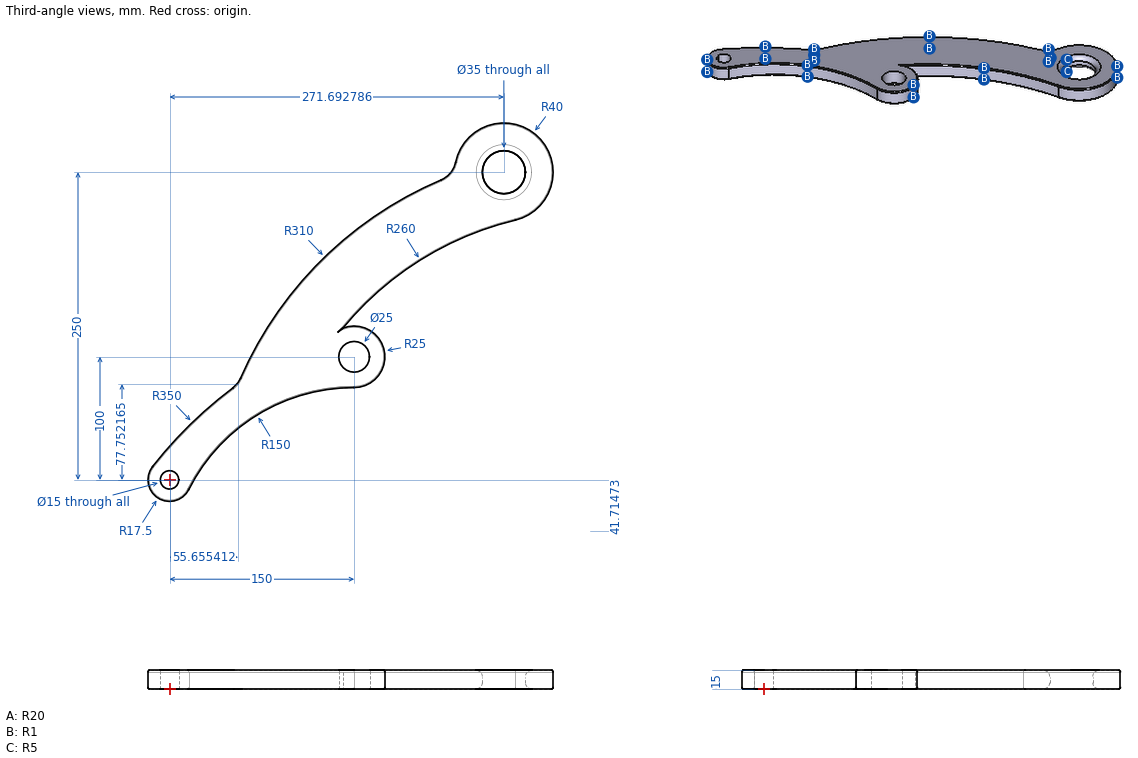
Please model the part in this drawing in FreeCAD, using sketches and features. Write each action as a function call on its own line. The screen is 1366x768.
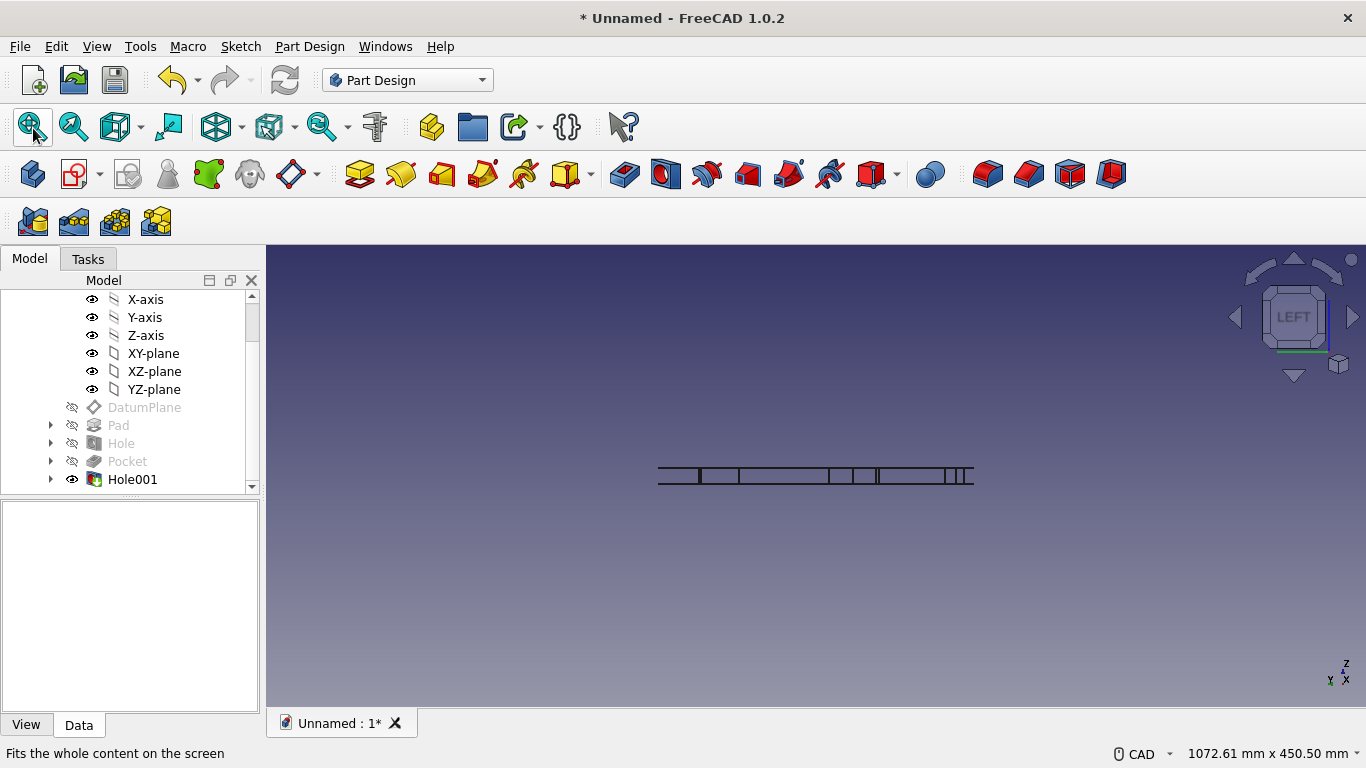
key(0)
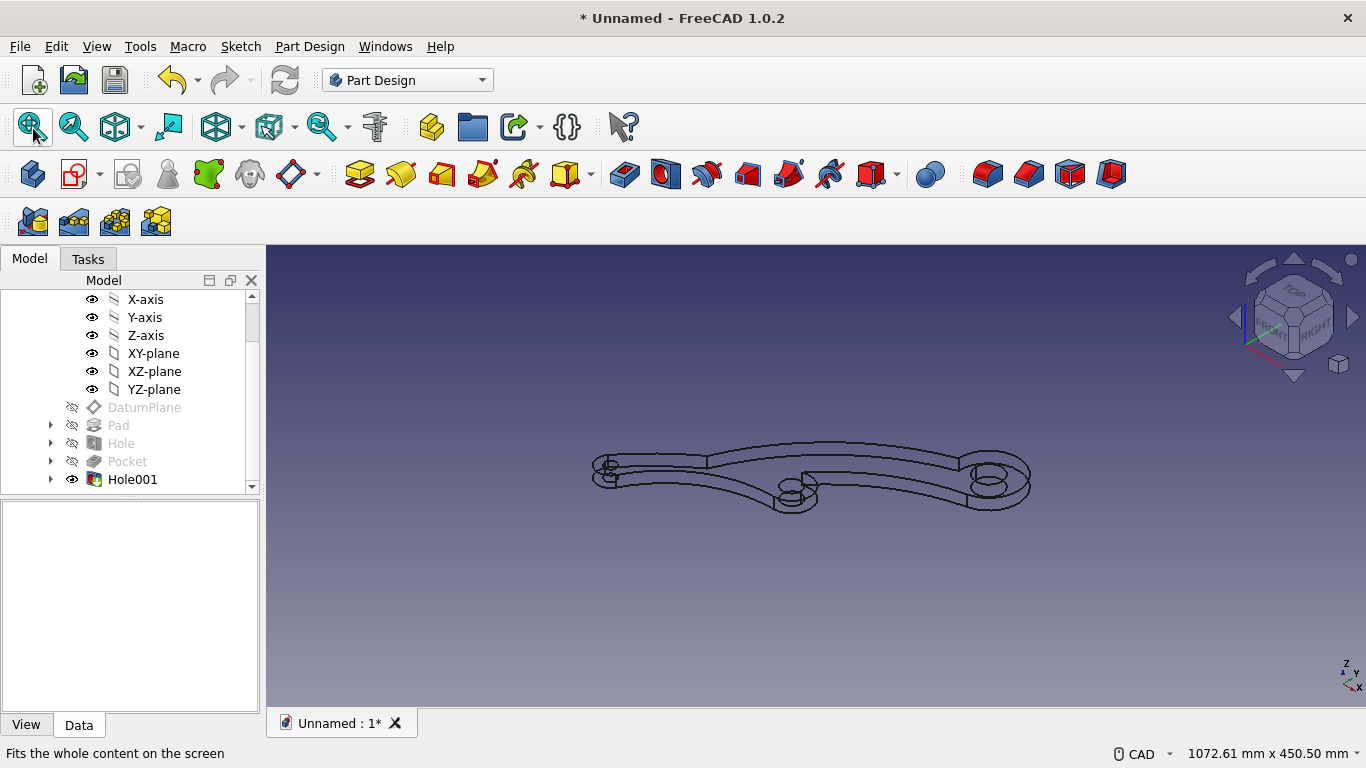
click(707, 461)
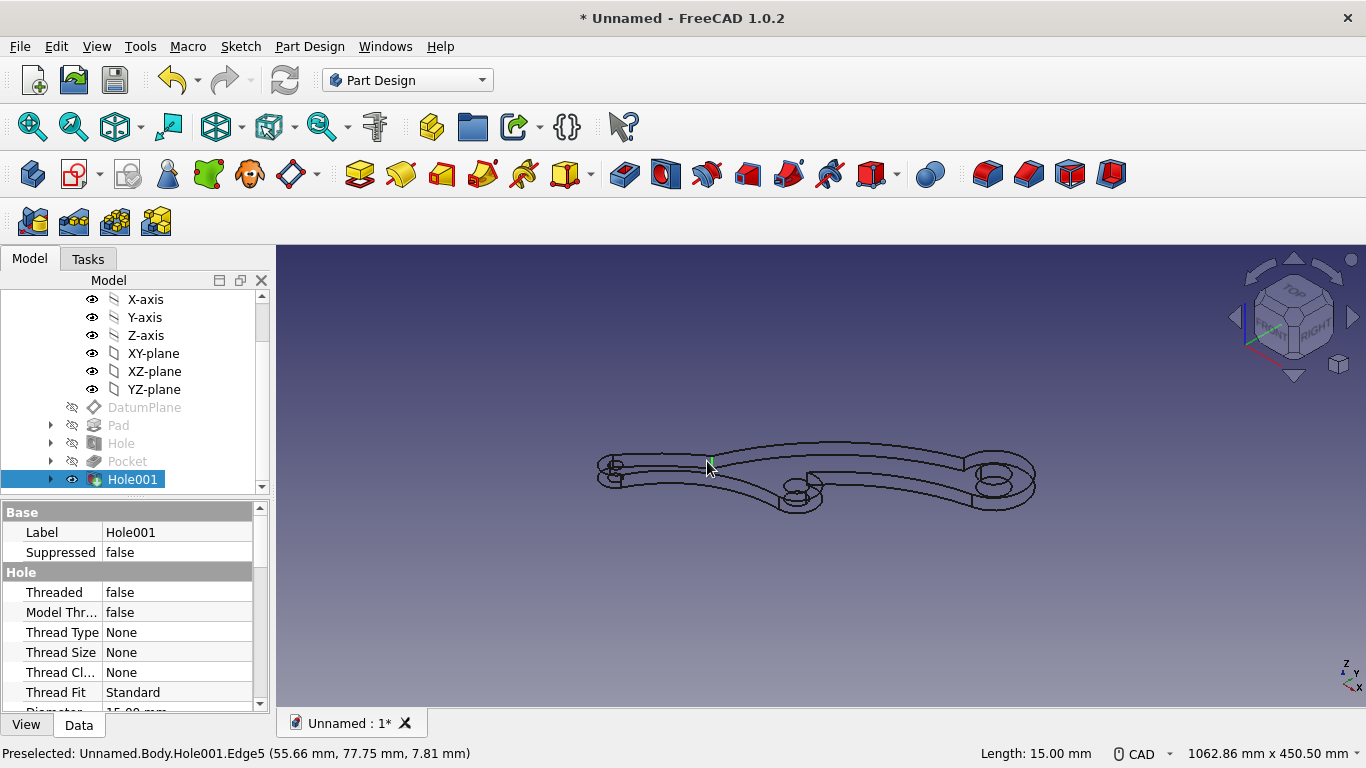
click(964, 464, ctrl)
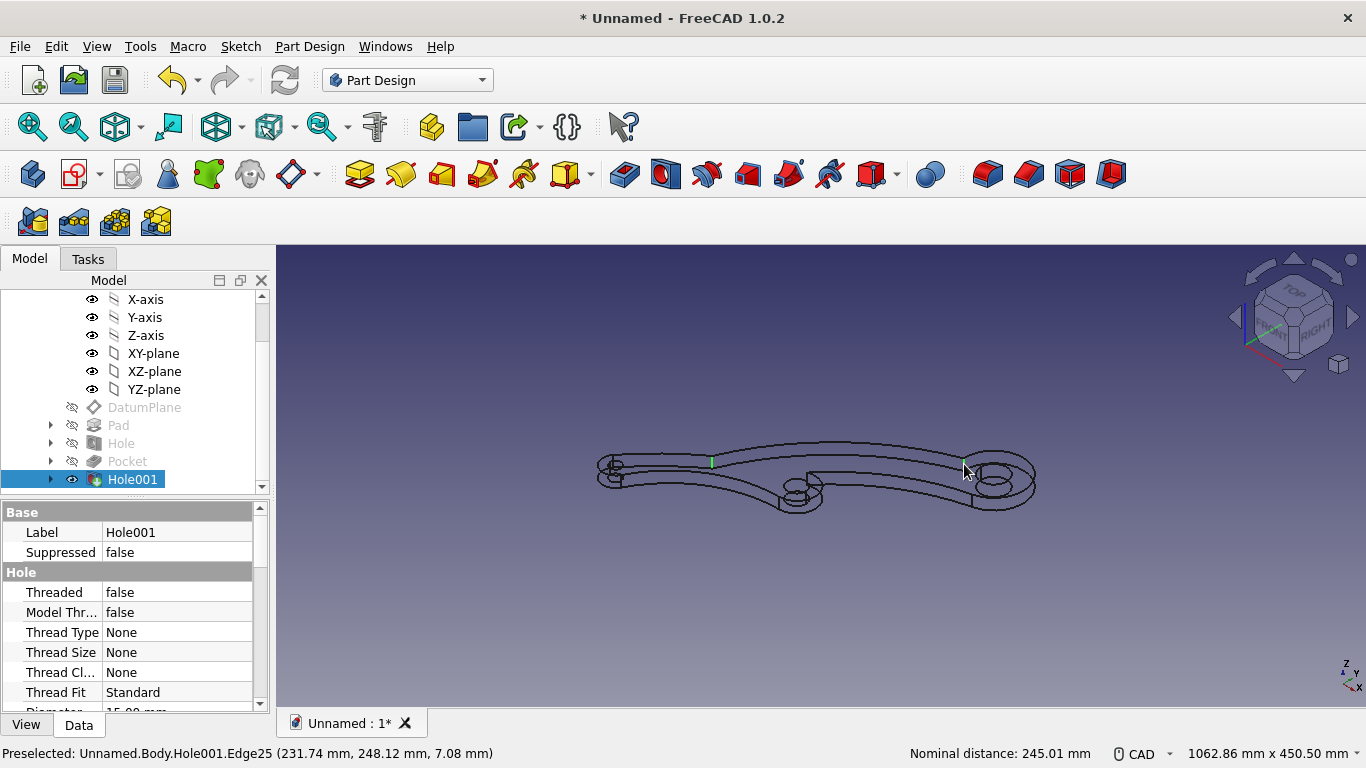
key(v)
key(1)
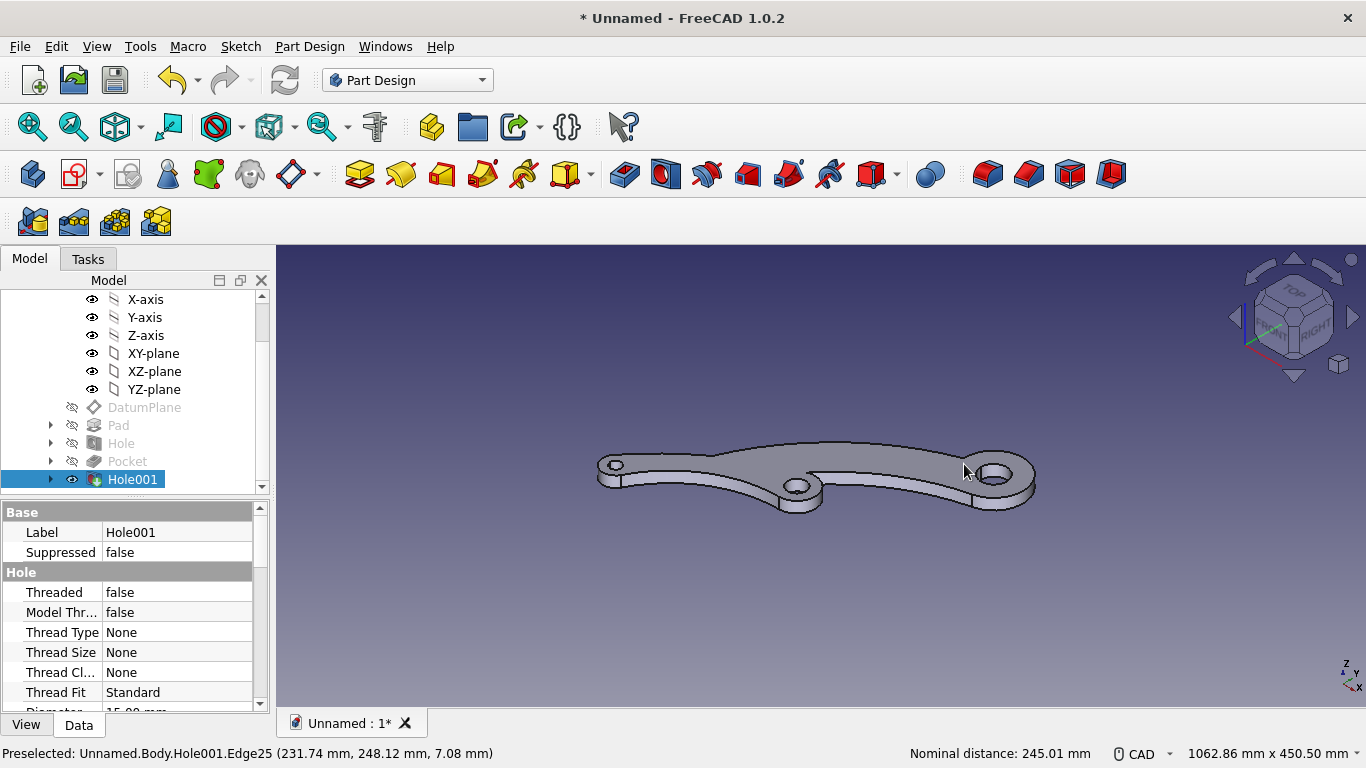
click(988, 174)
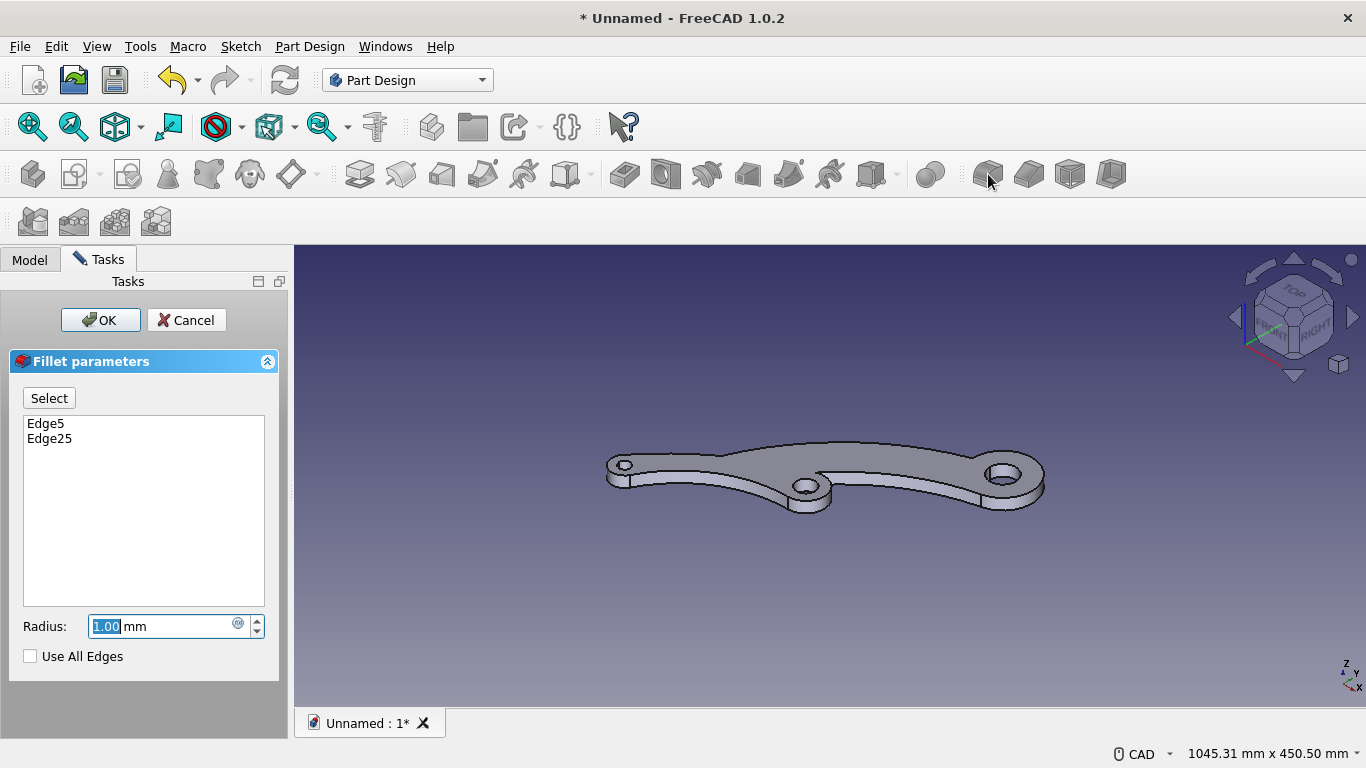
text(20)
key(Tab)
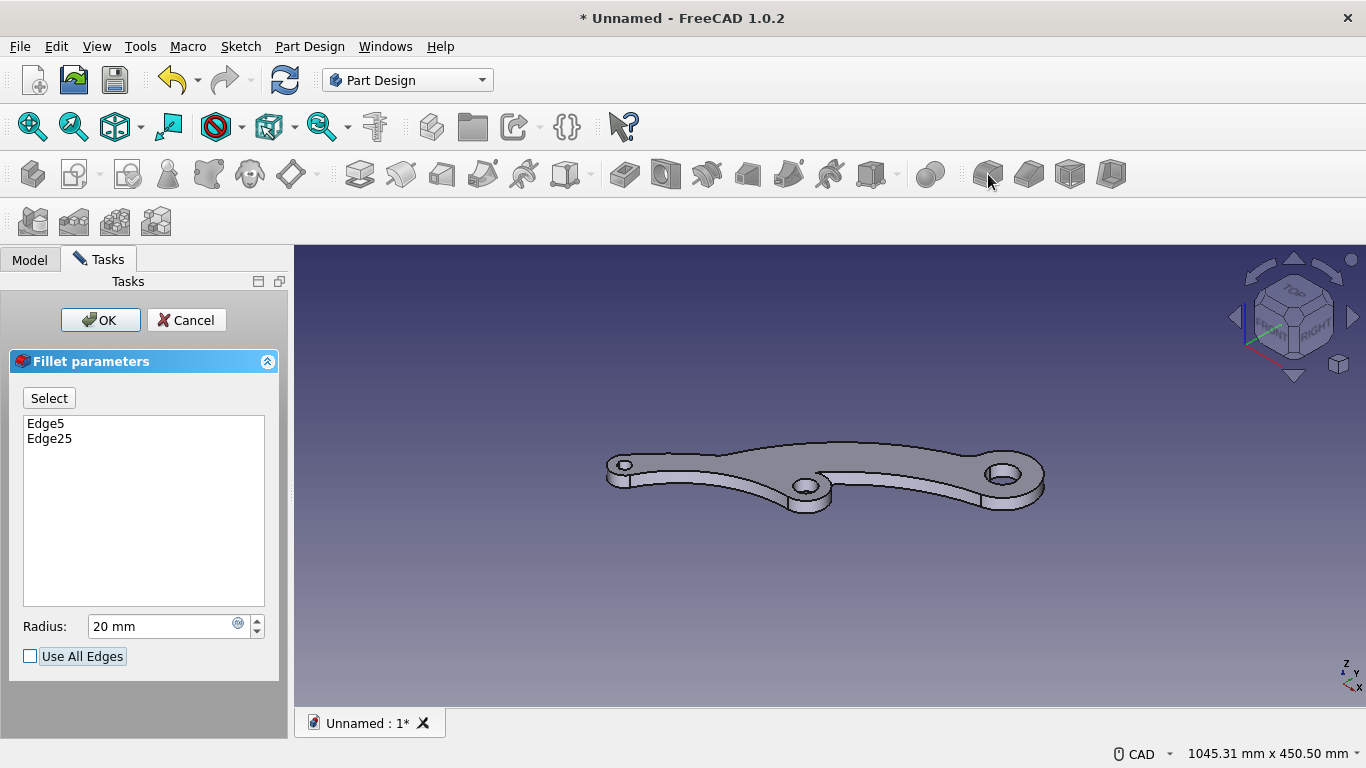
click(101, 320)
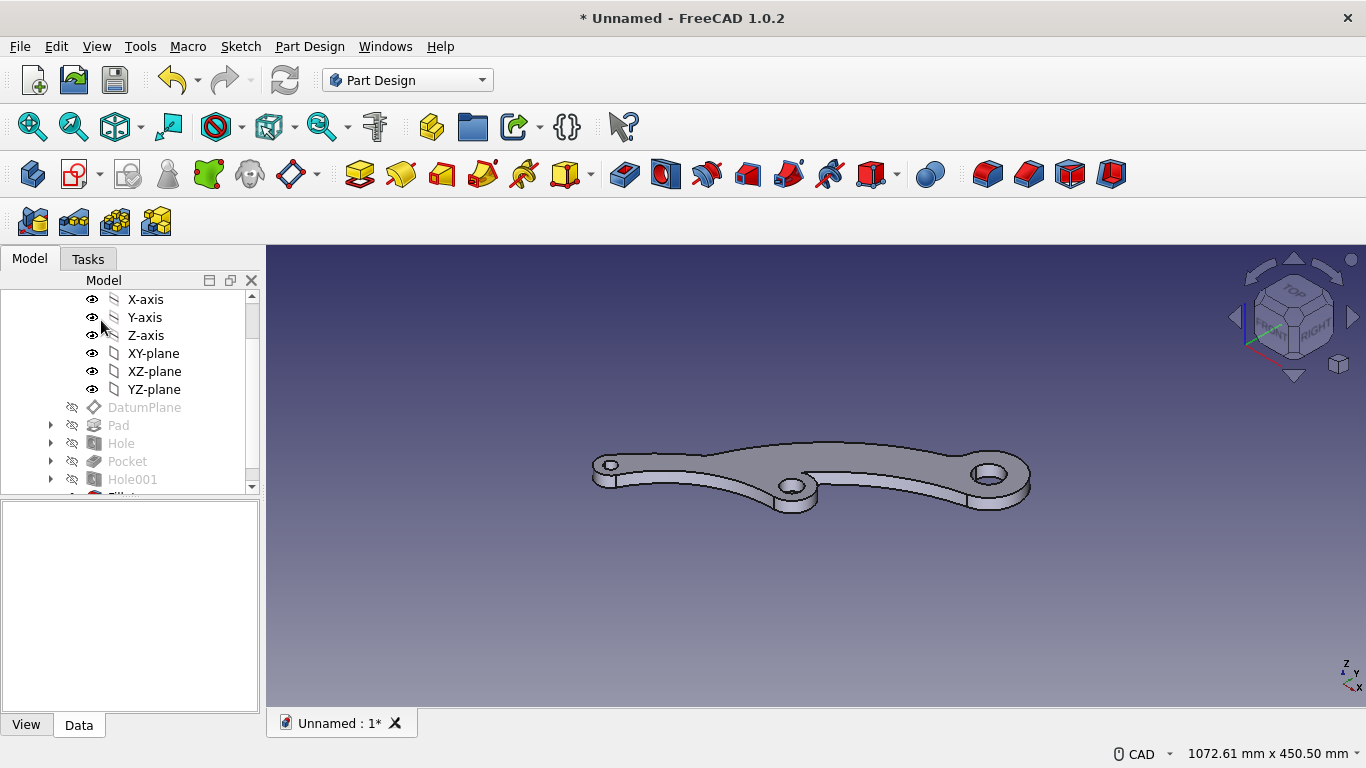
click(1026, 483)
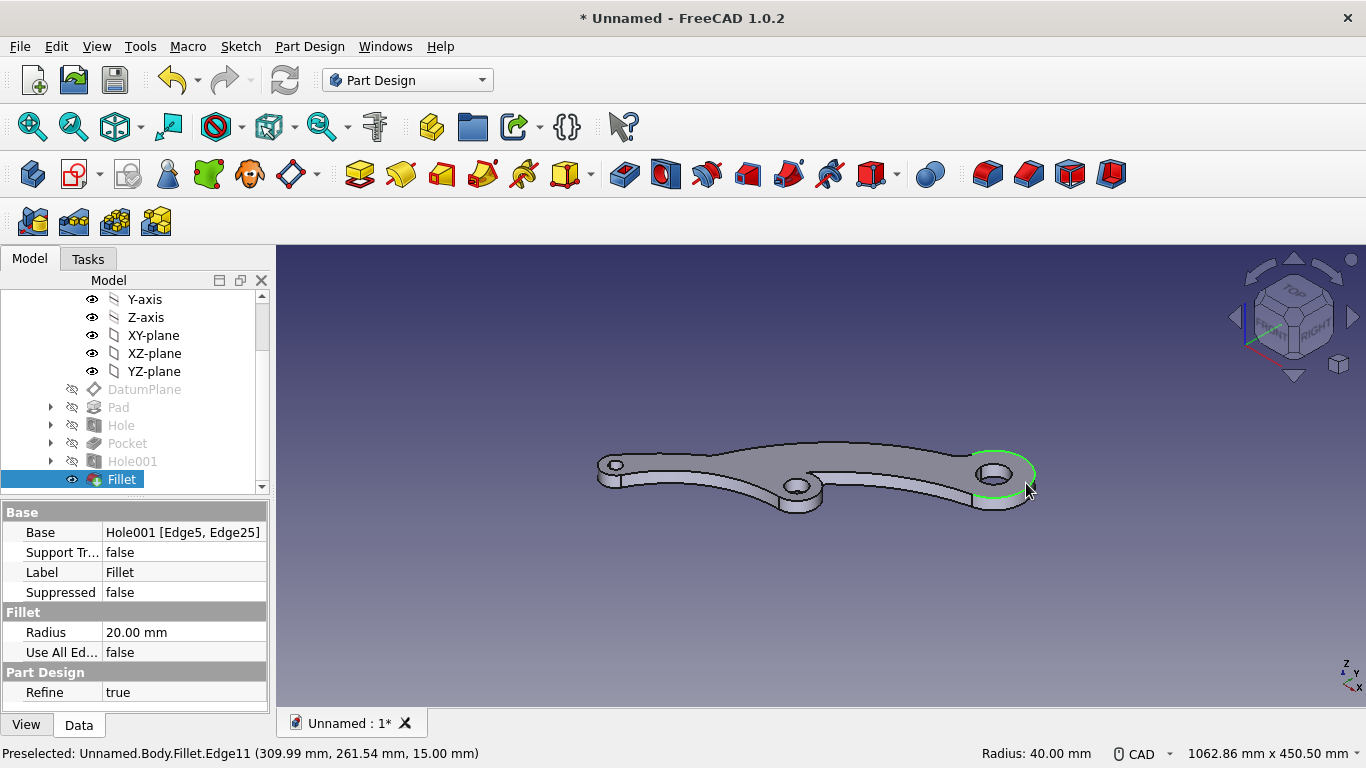
click(604, 485, ctrl)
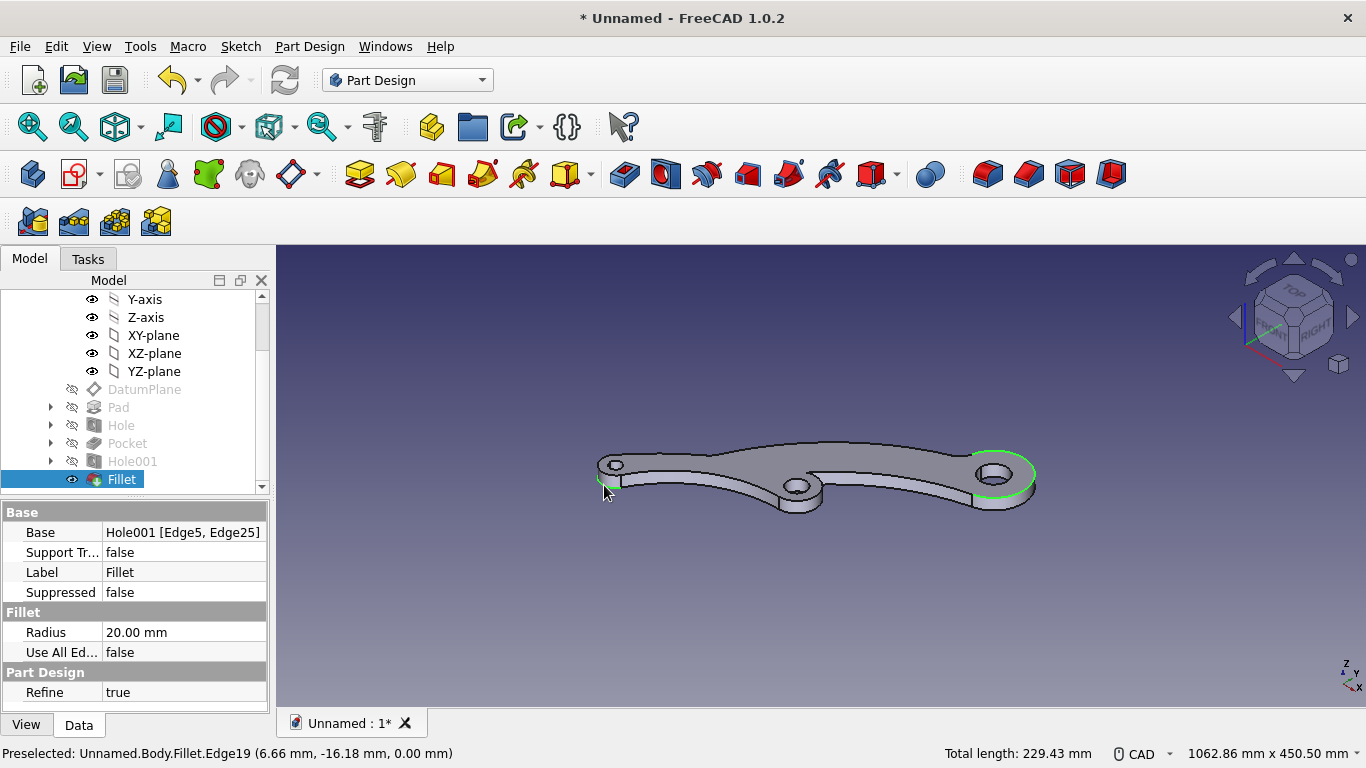
click(893, 475, ctrl)